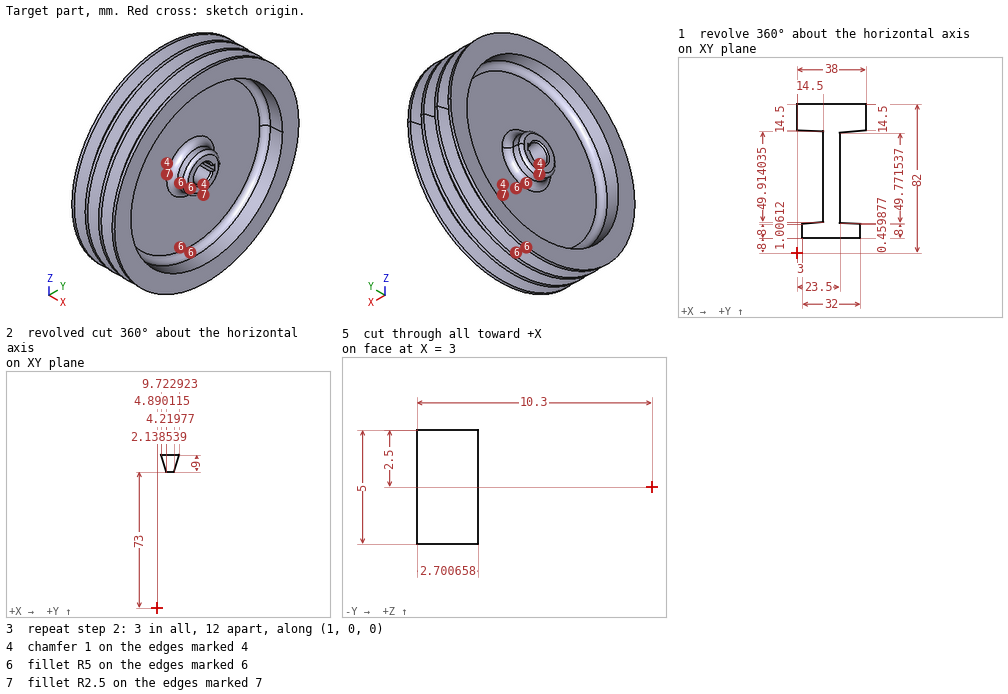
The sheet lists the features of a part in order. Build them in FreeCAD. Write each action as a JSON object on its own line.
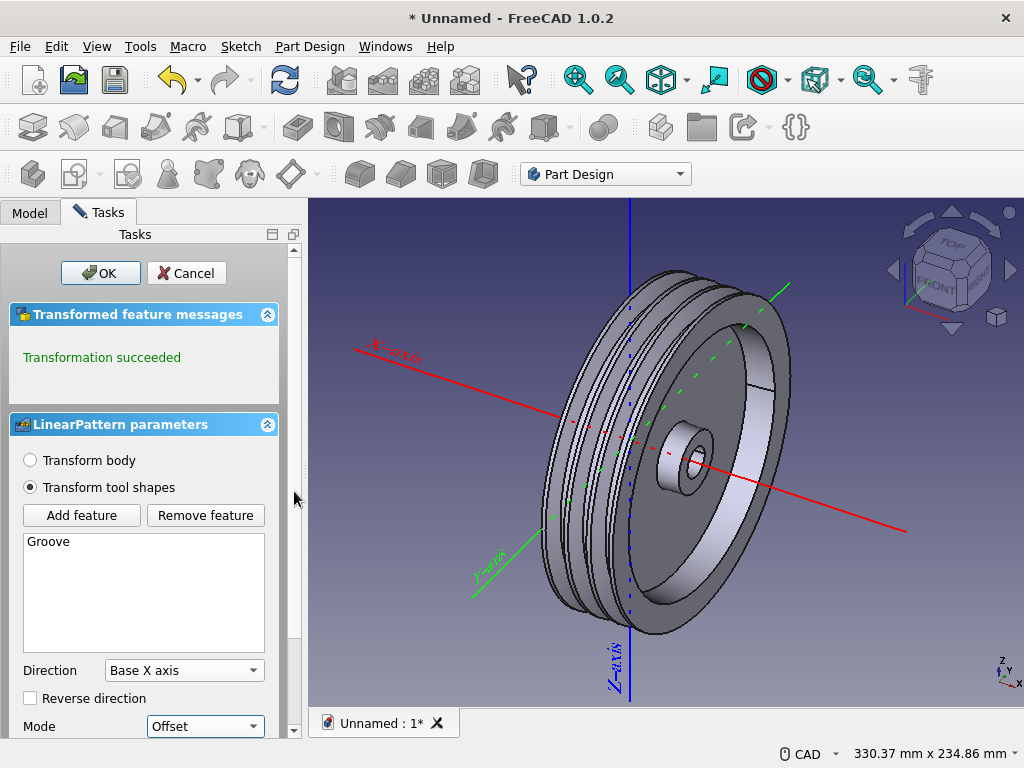
{"action": "left_click", "coordinate": [101, 273]}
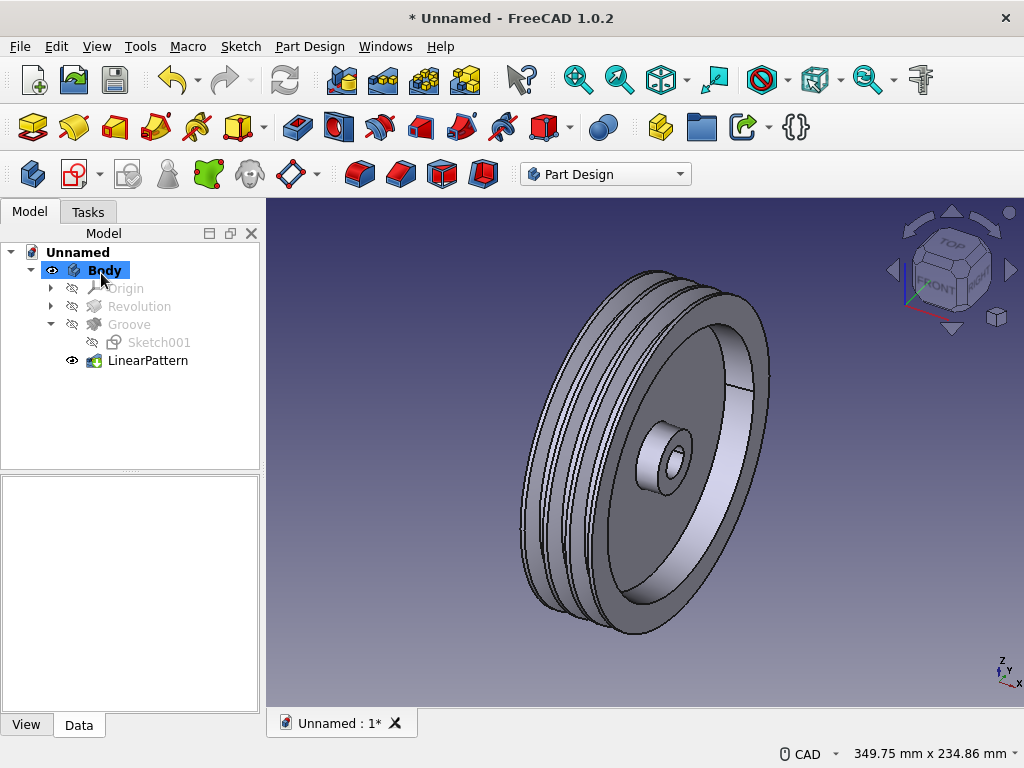
{"action": "left_click", "coordinate": [668, 477]}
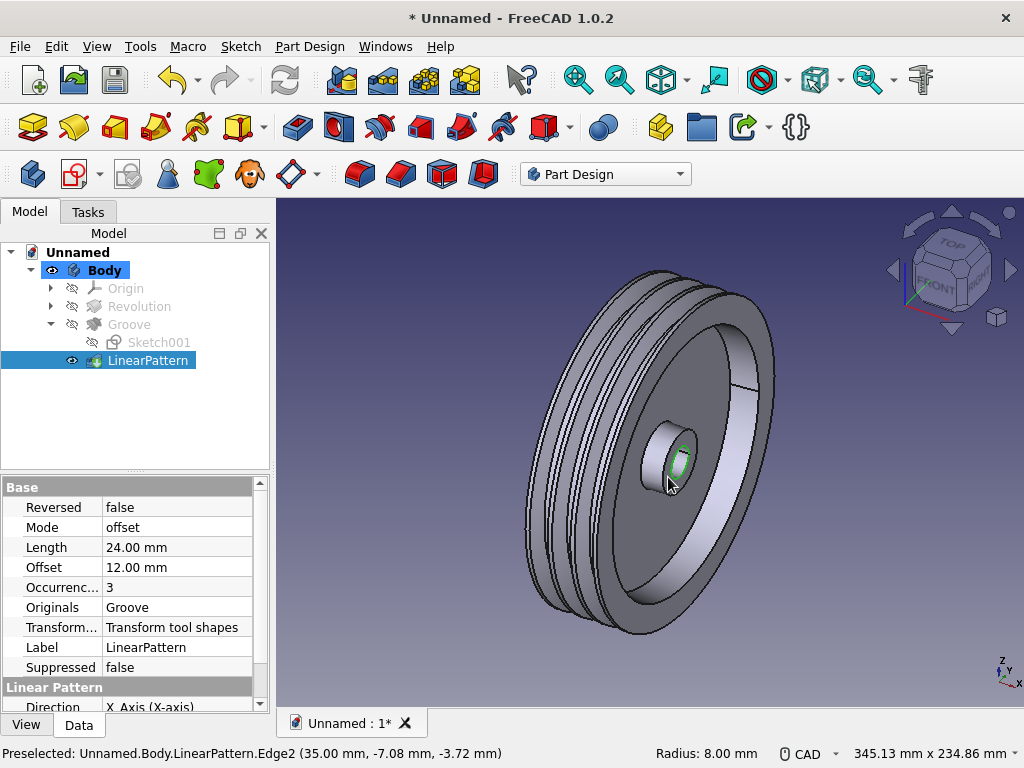
{"action": "key", "text": "0"}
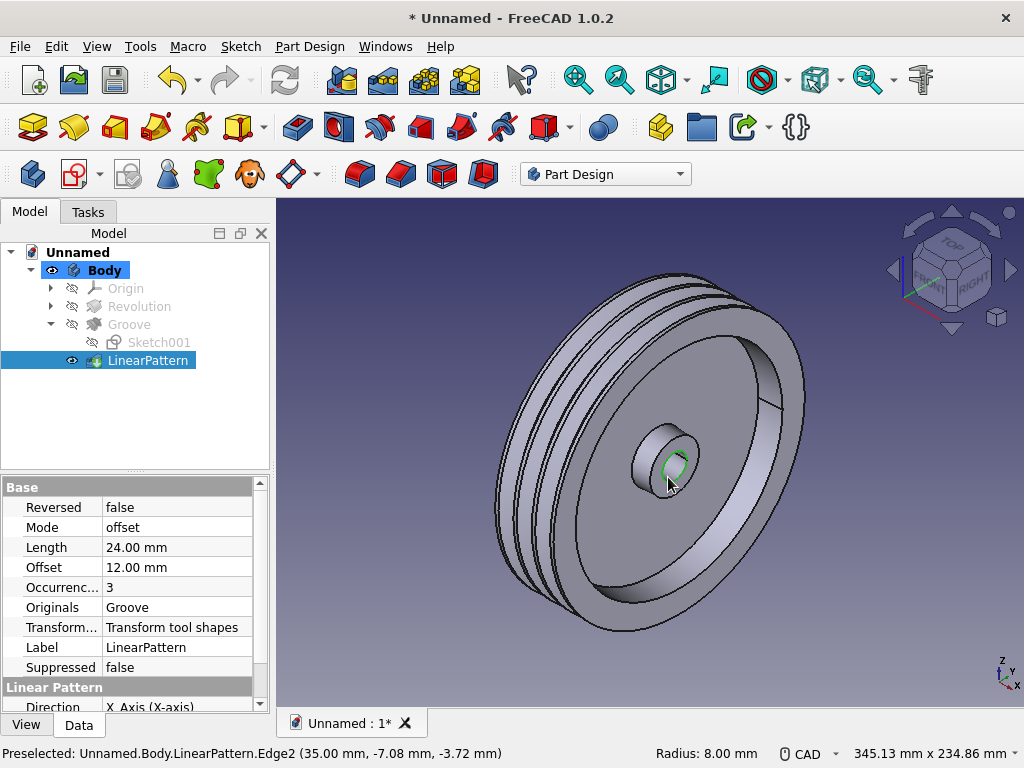
{"action": "key", "text": "2"}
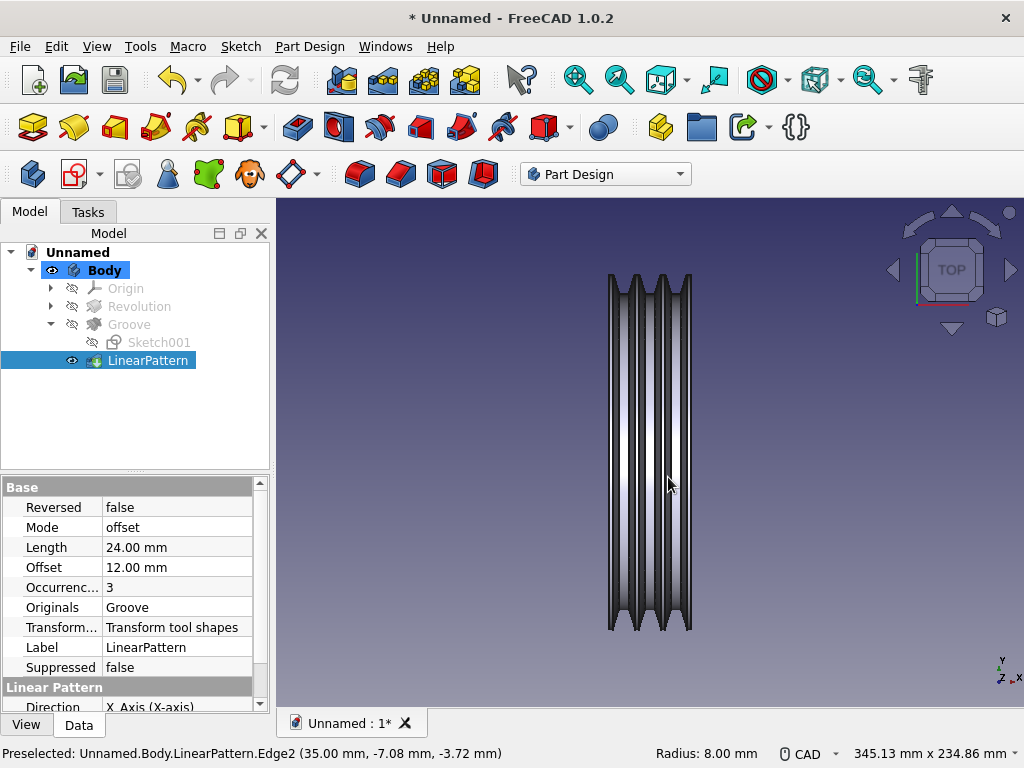
{"action": "key", "text": "1"}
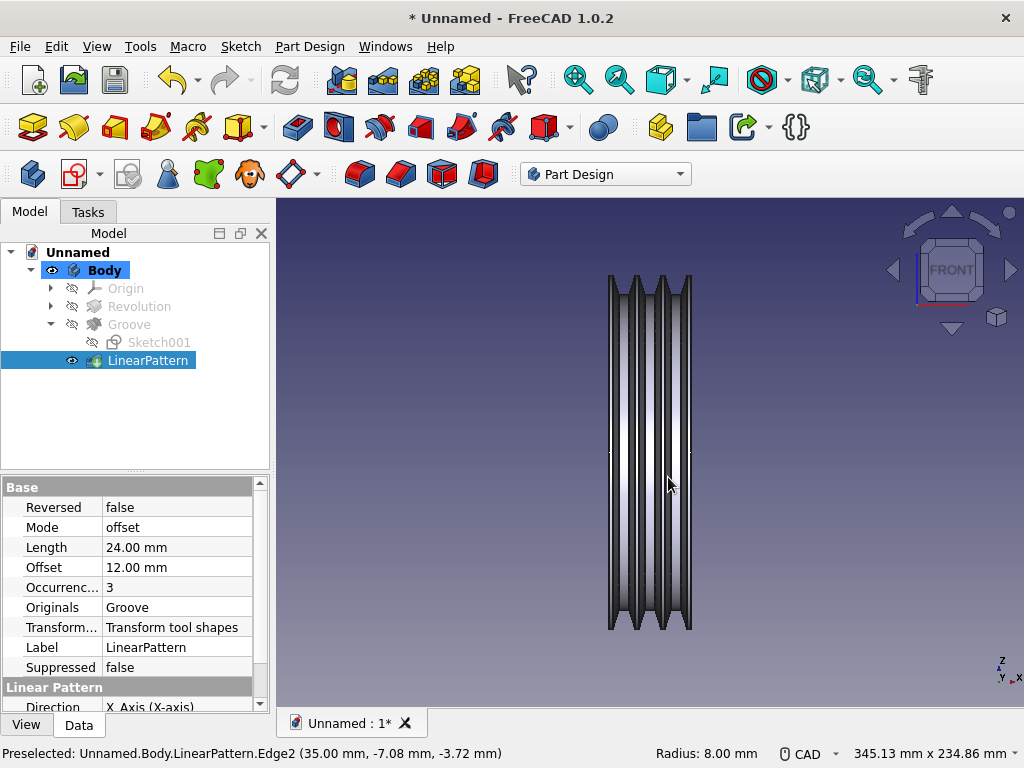
{"action": "key", "text": "3"}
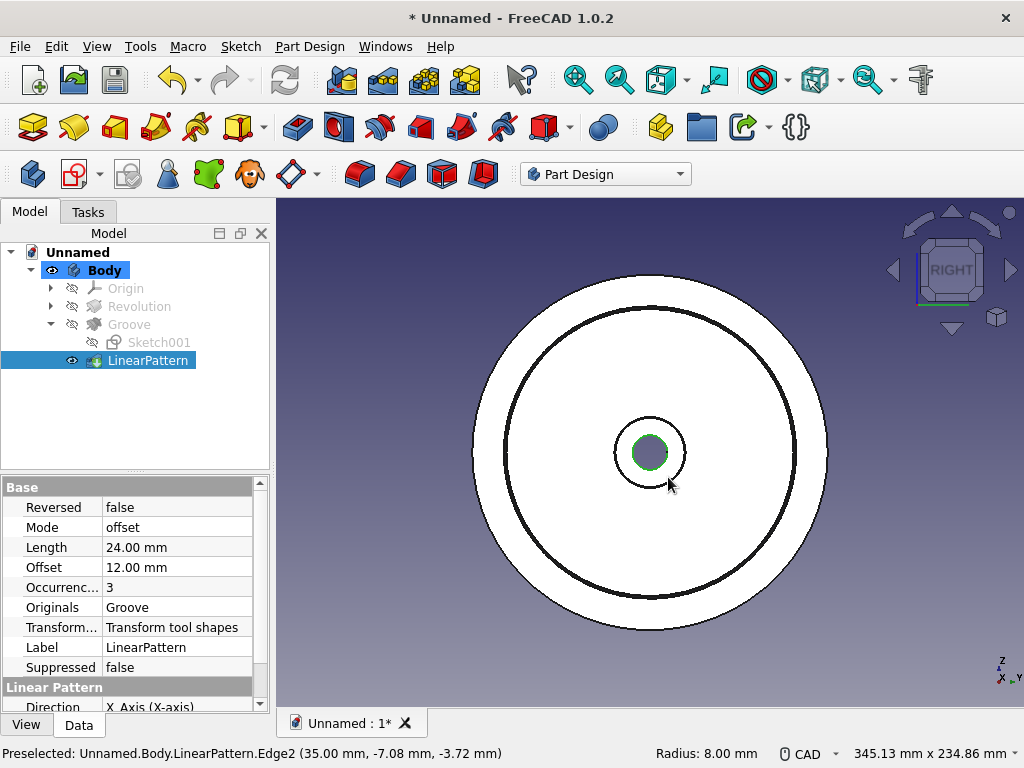
{"action": "key", "text": "5"}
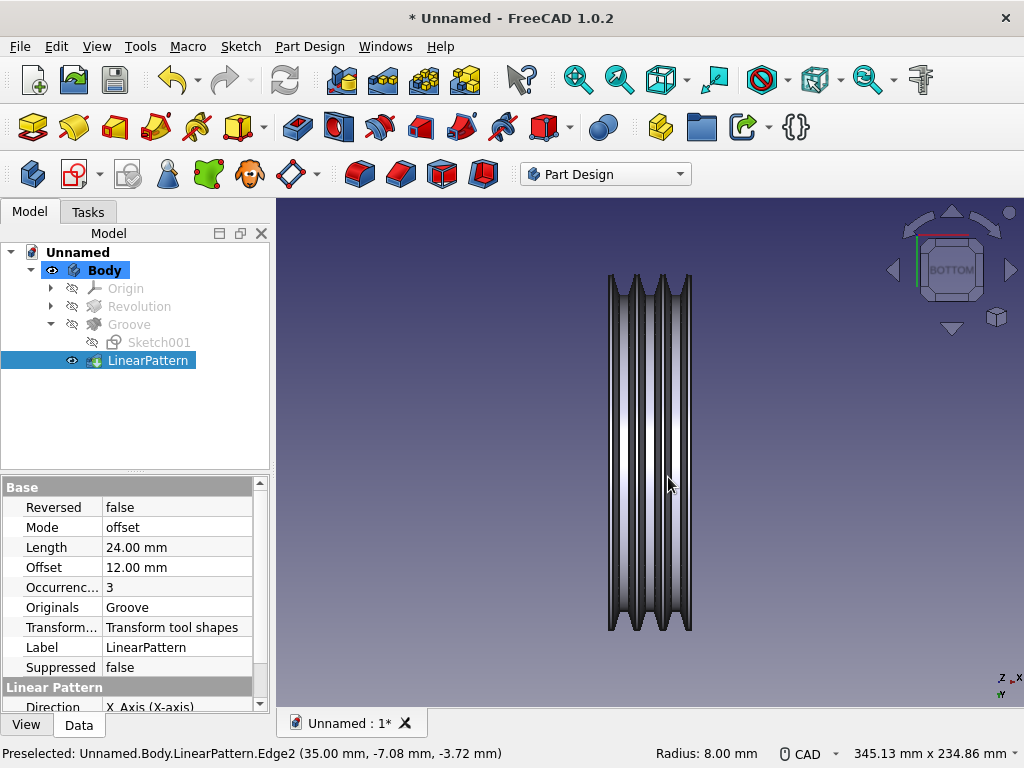
{"action": "key", "text": "4"}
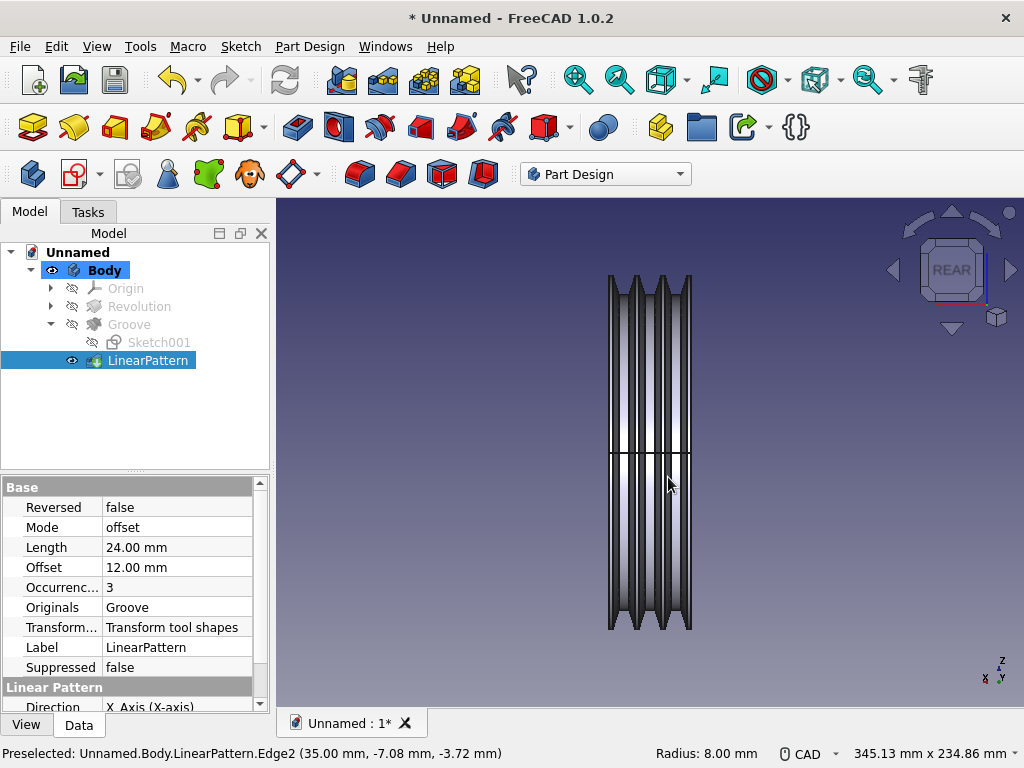
{"action": "key", "text": "6"}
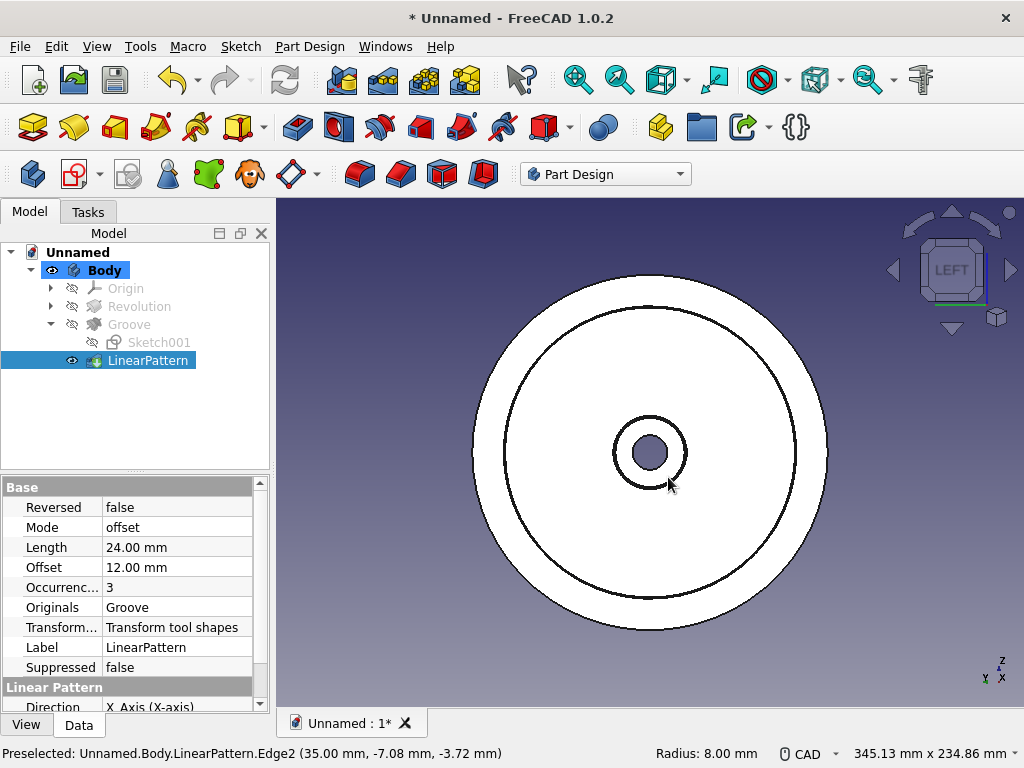
{"action": "left_click", "coordinate": [667, 451], "text": "ctrl"}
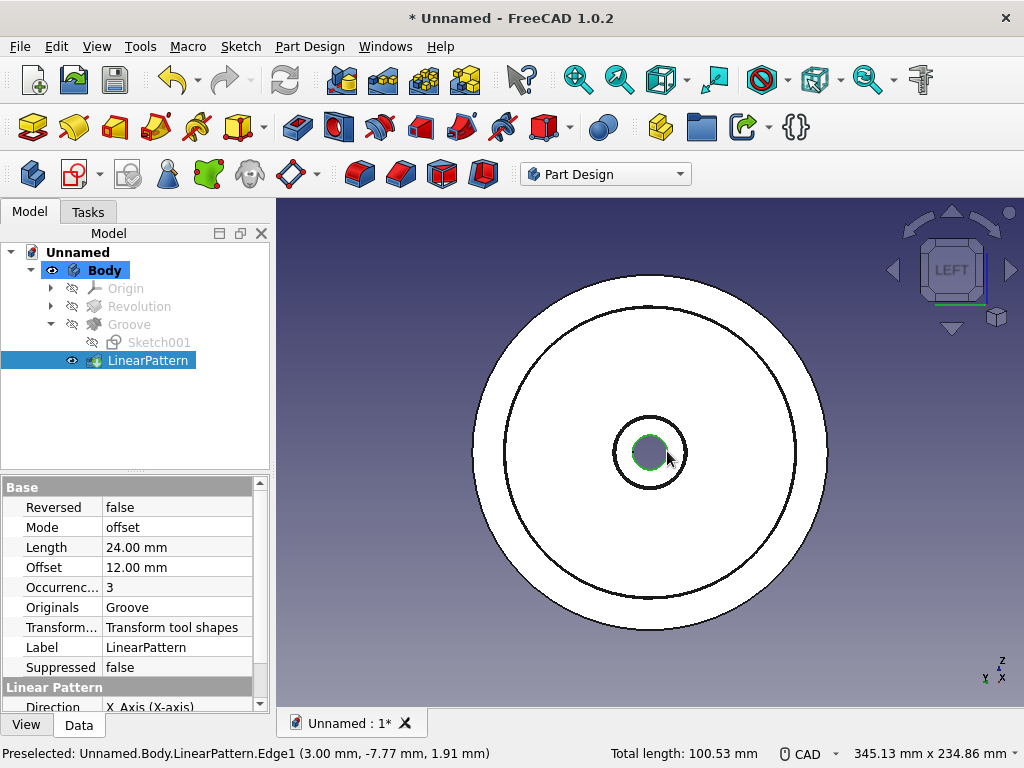
{"action": "left_click", "coordinate": [401, 174]}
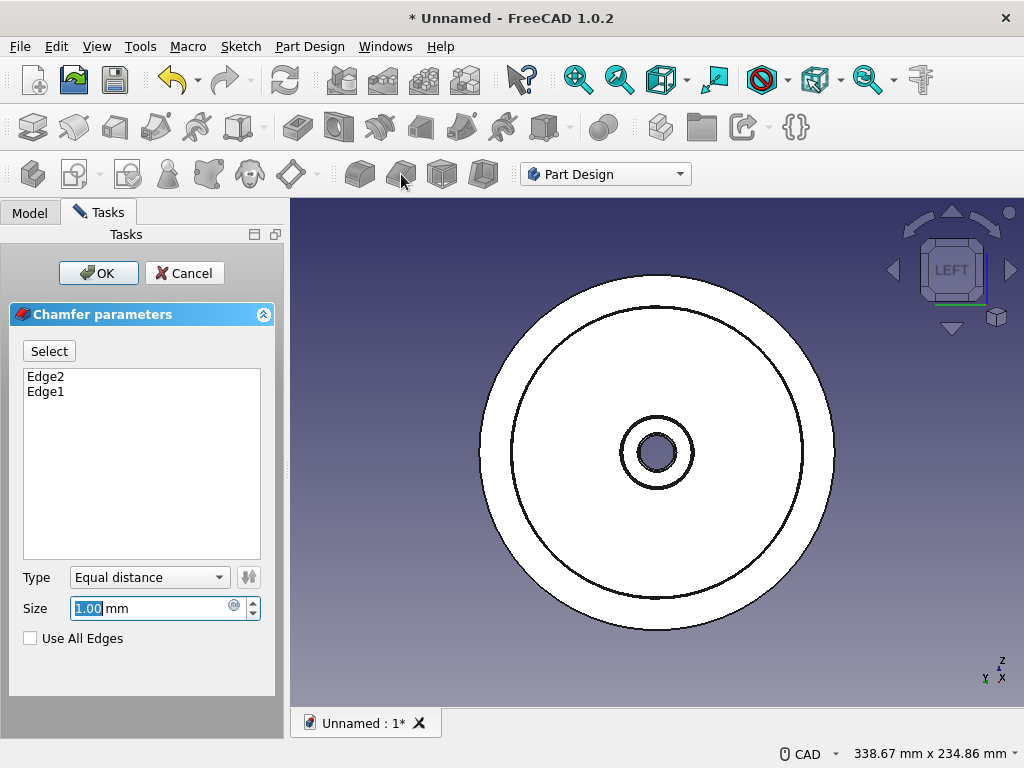
{"action": "type", "text": "1"}
{"action": "key", "text": "Tab"}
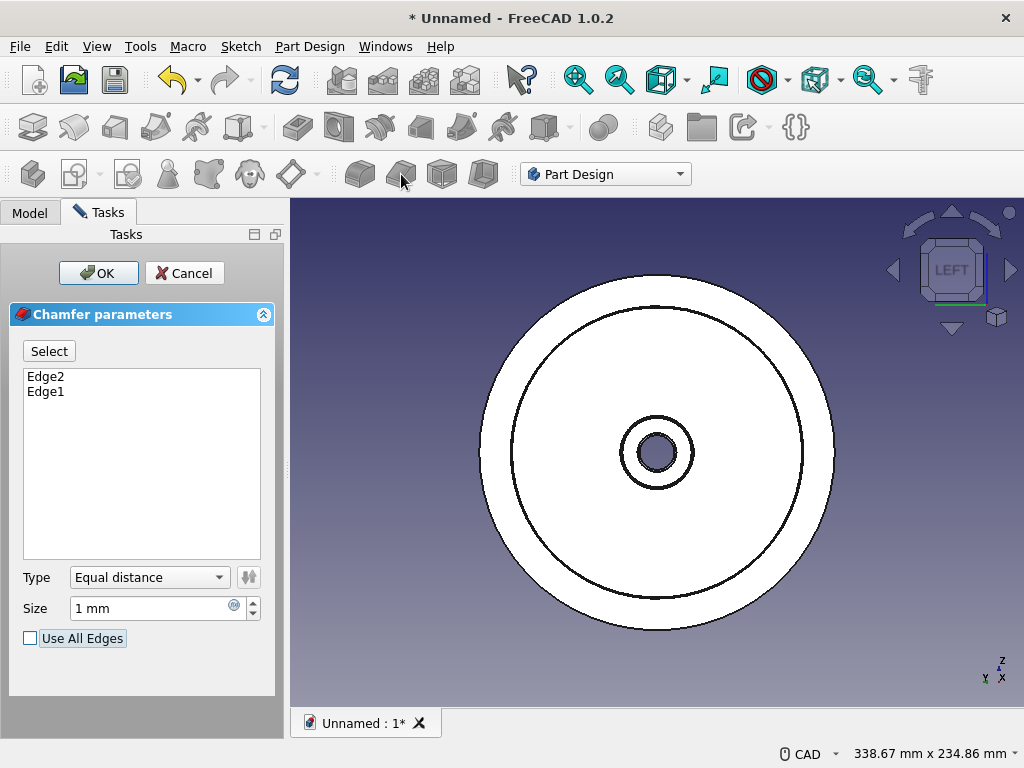
{"action": "left_click", "coordinate": [99, 273]}